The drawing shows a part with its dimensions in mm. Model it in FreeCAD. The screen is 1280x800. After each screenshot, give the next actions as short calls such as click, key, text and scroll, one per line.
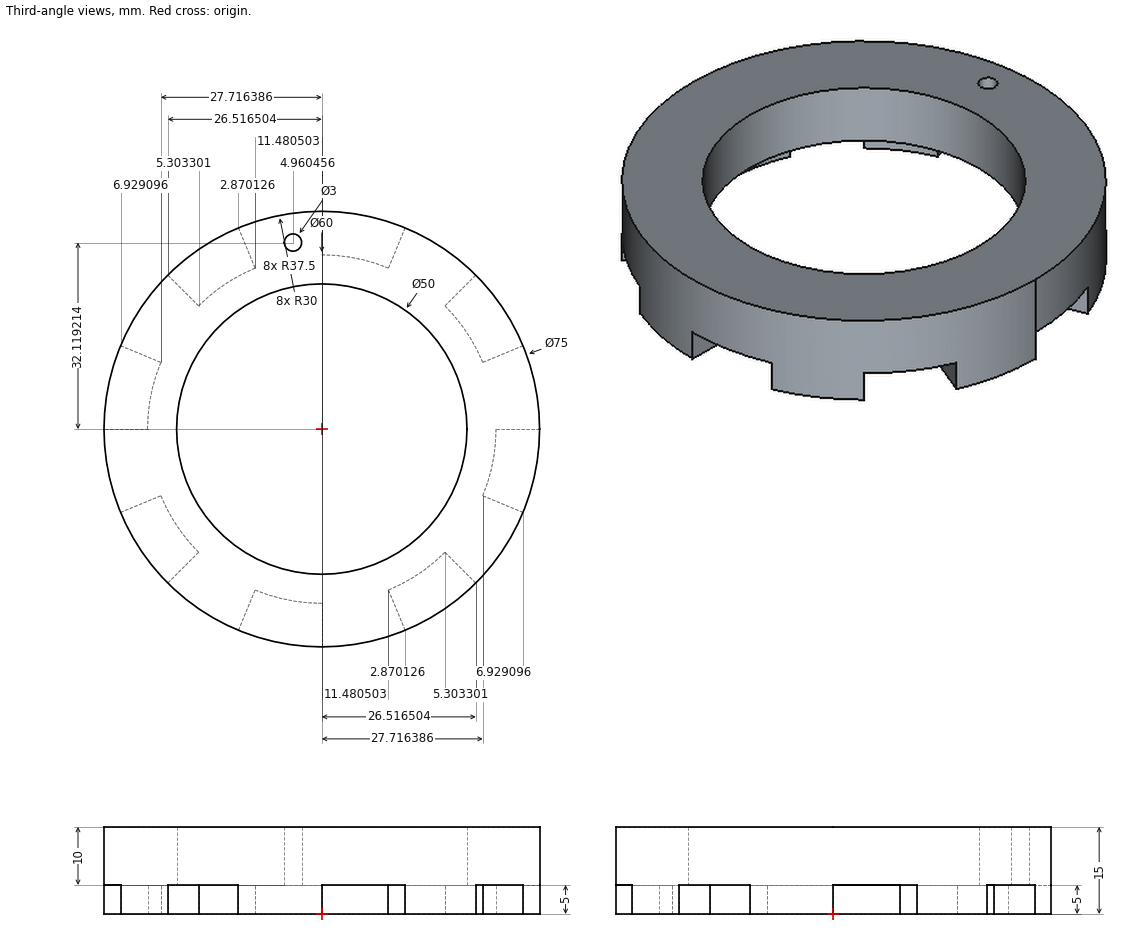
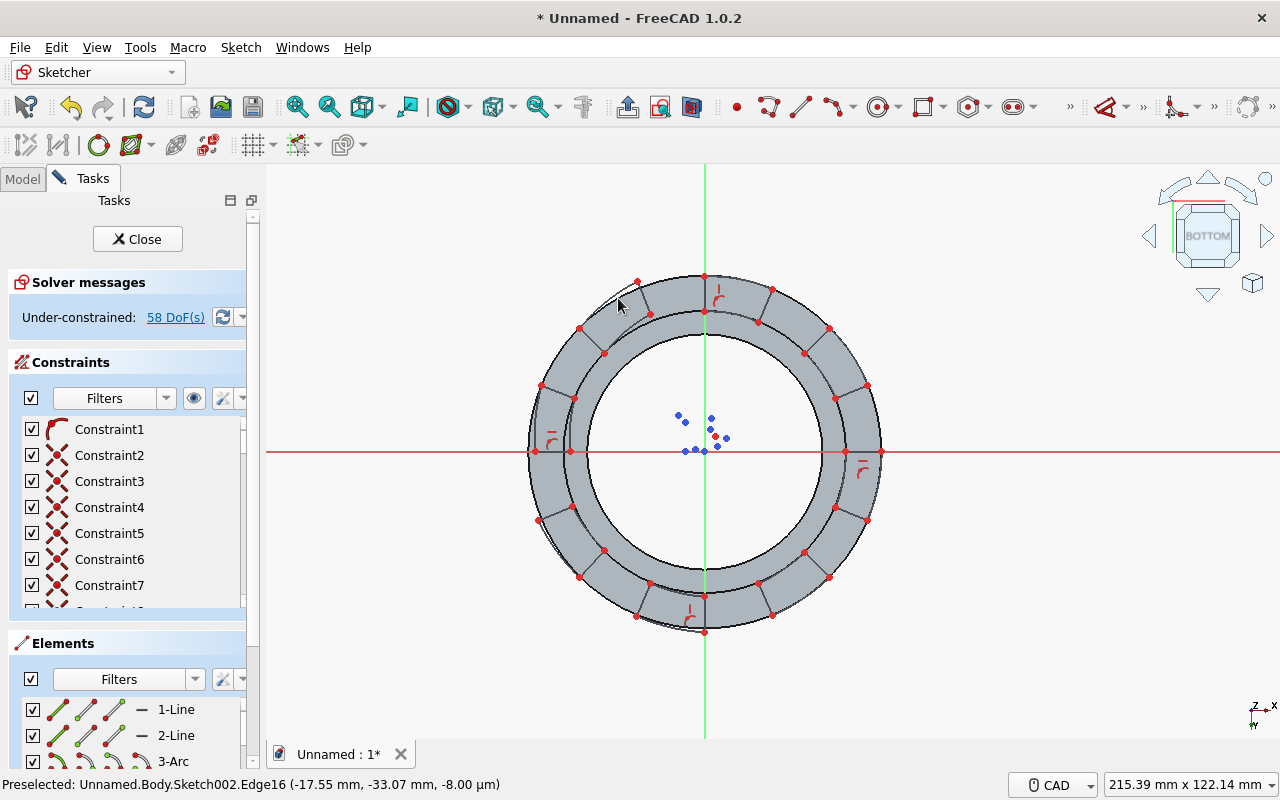
click(666, 589)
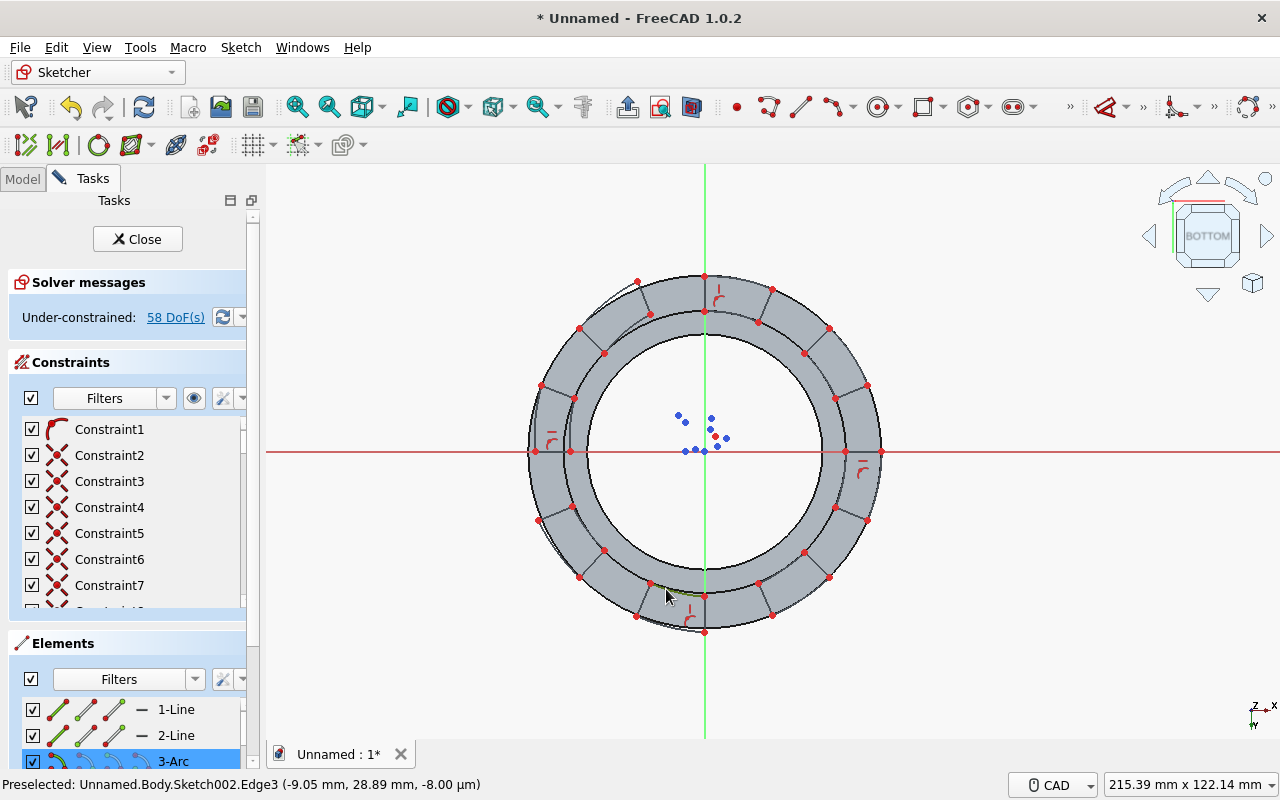
click(743, 316)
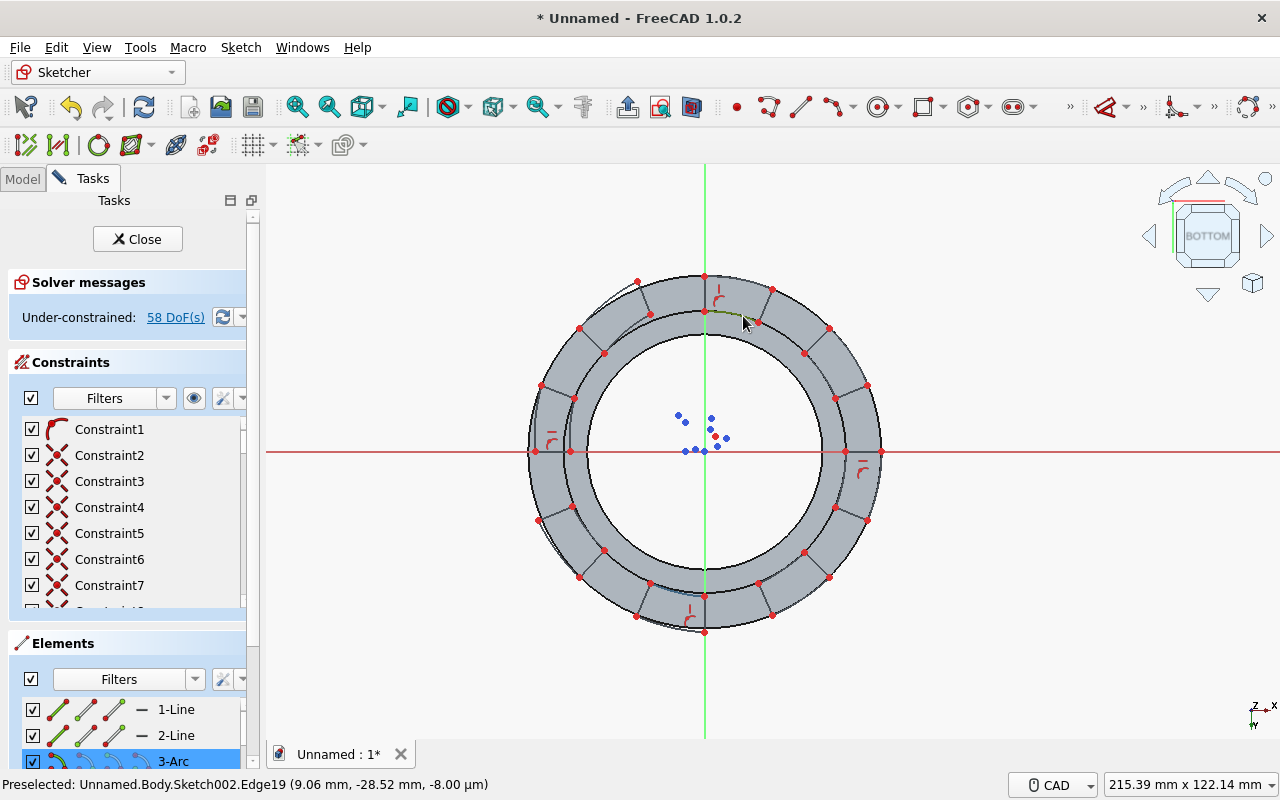
key(c)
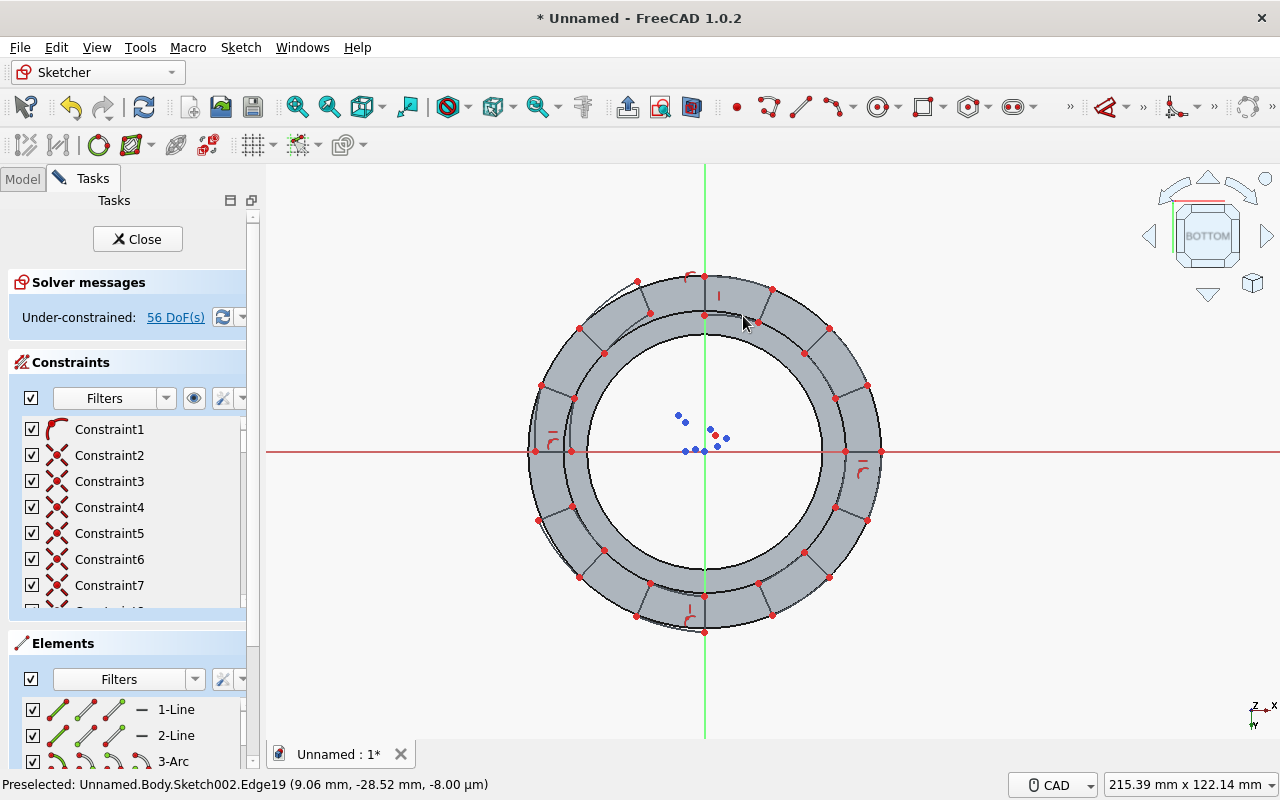
click(666, 589)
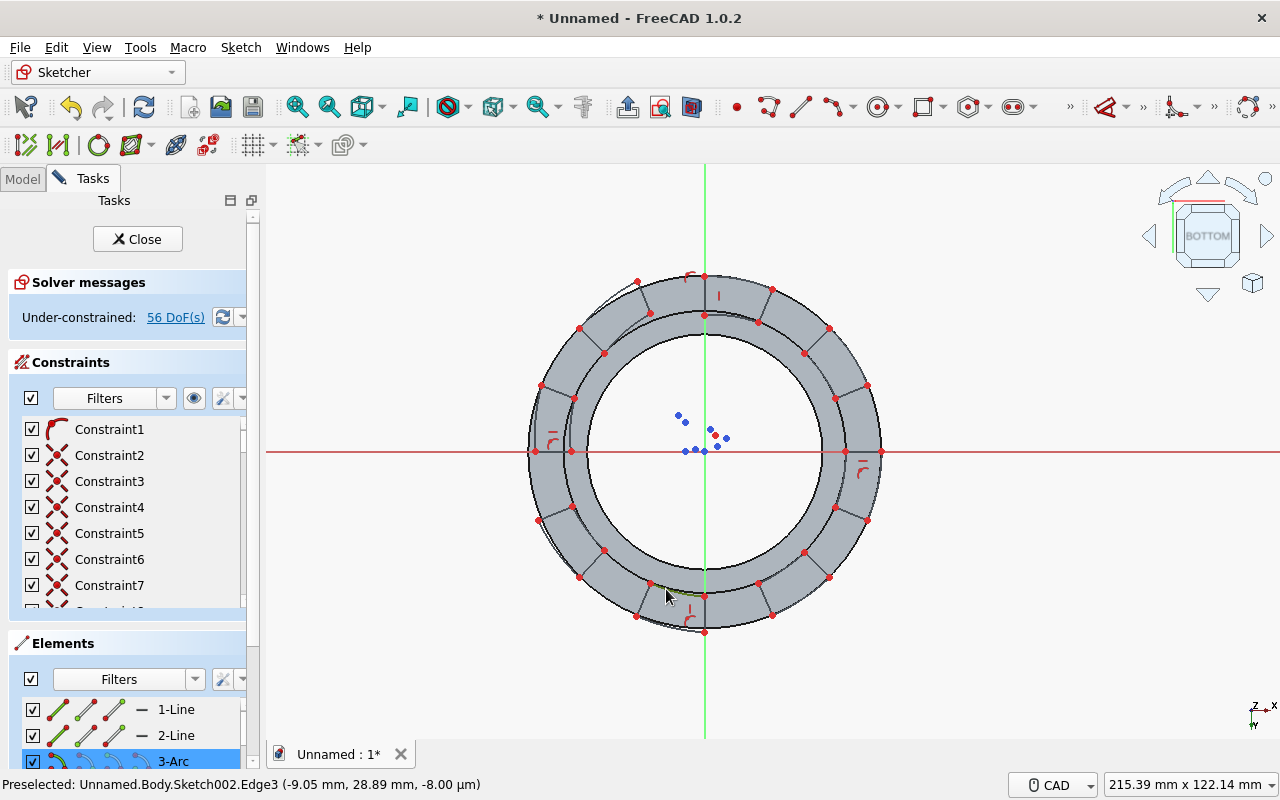
click(753, 282)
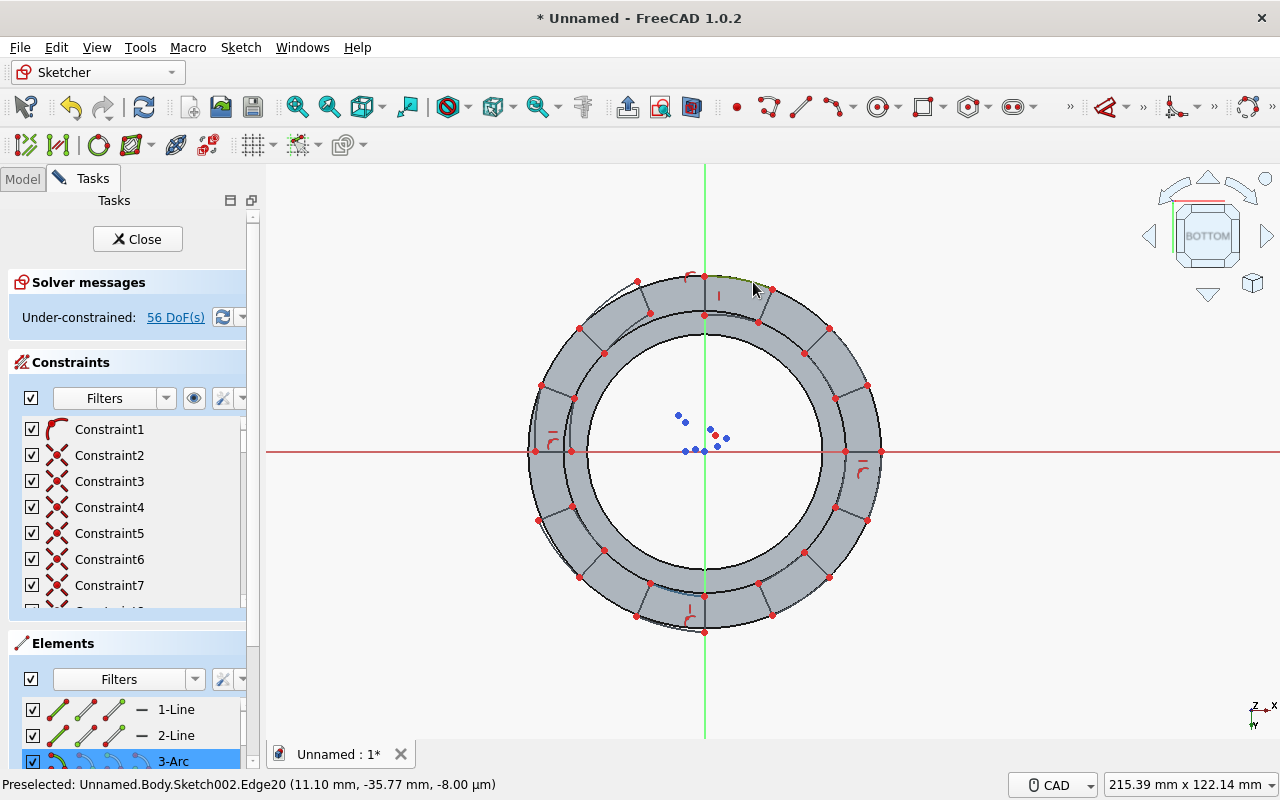
key(c)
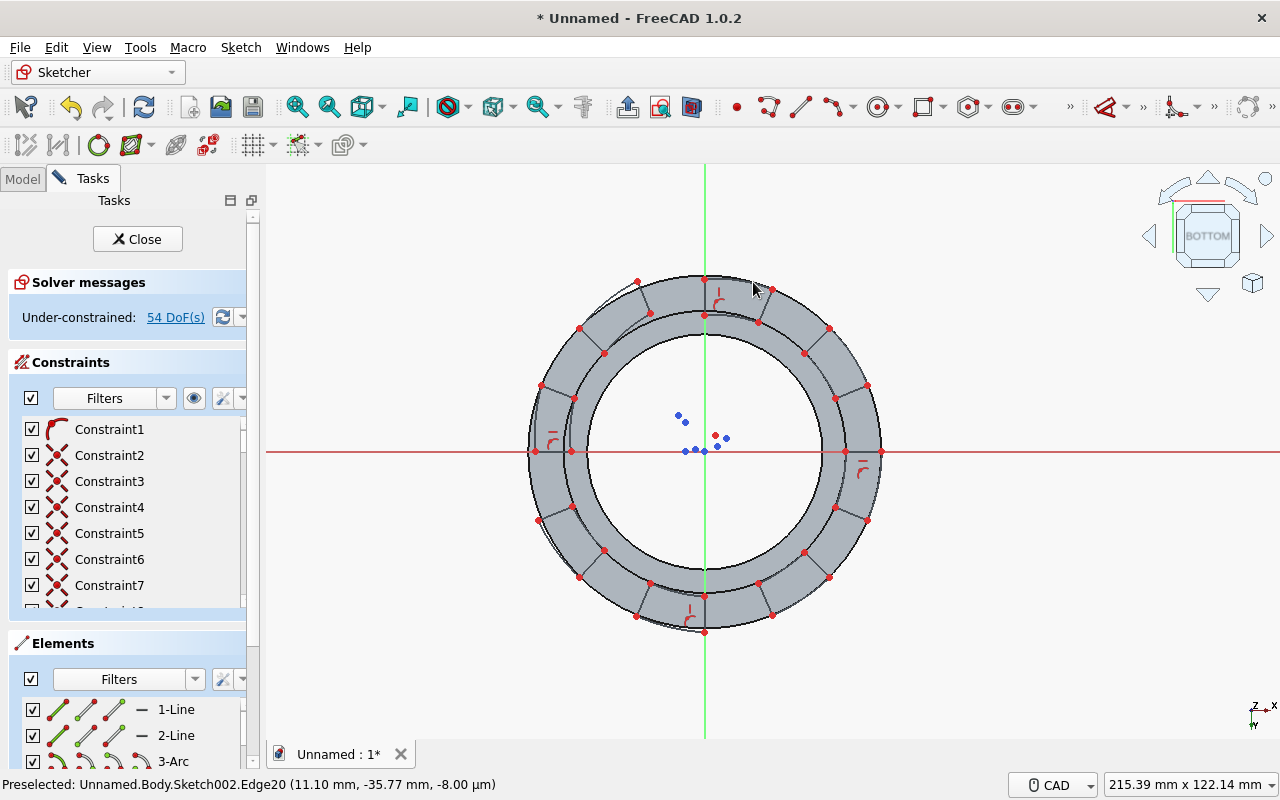
click(666, 589)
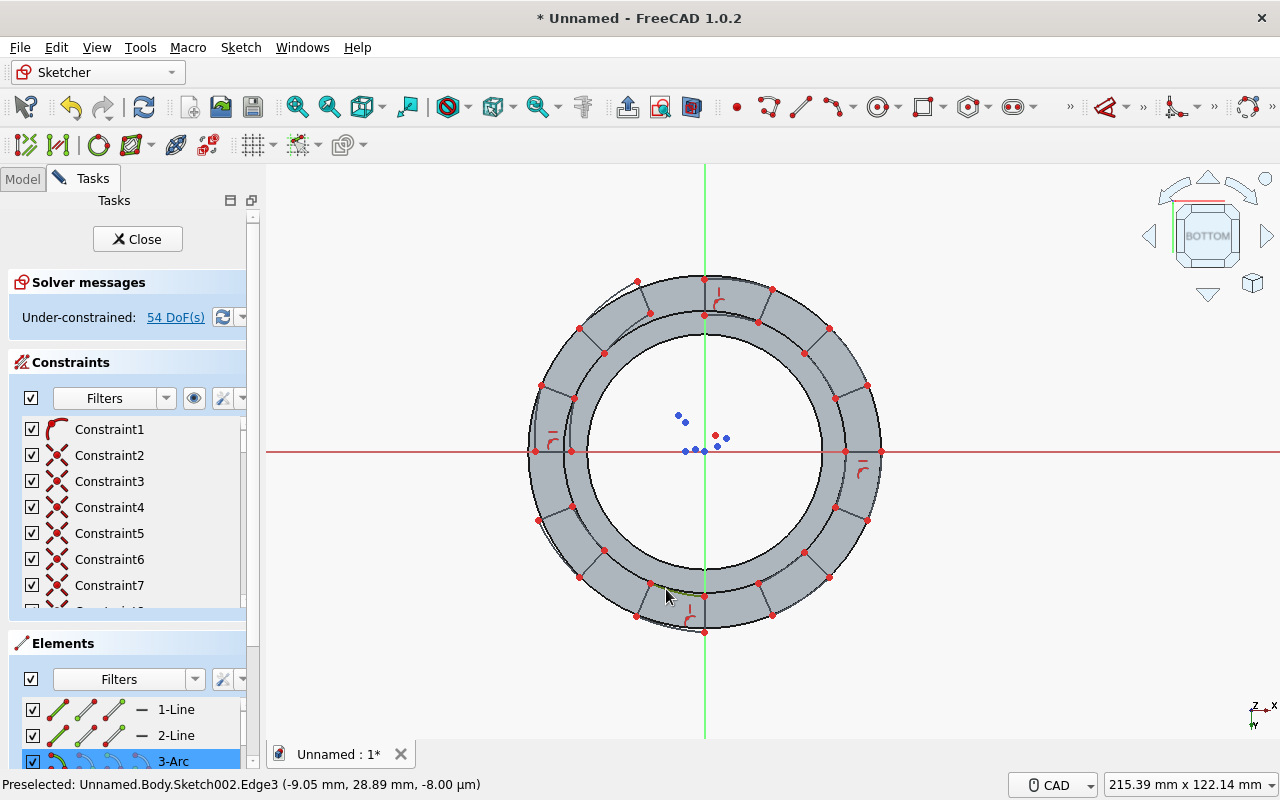
click(828, 384)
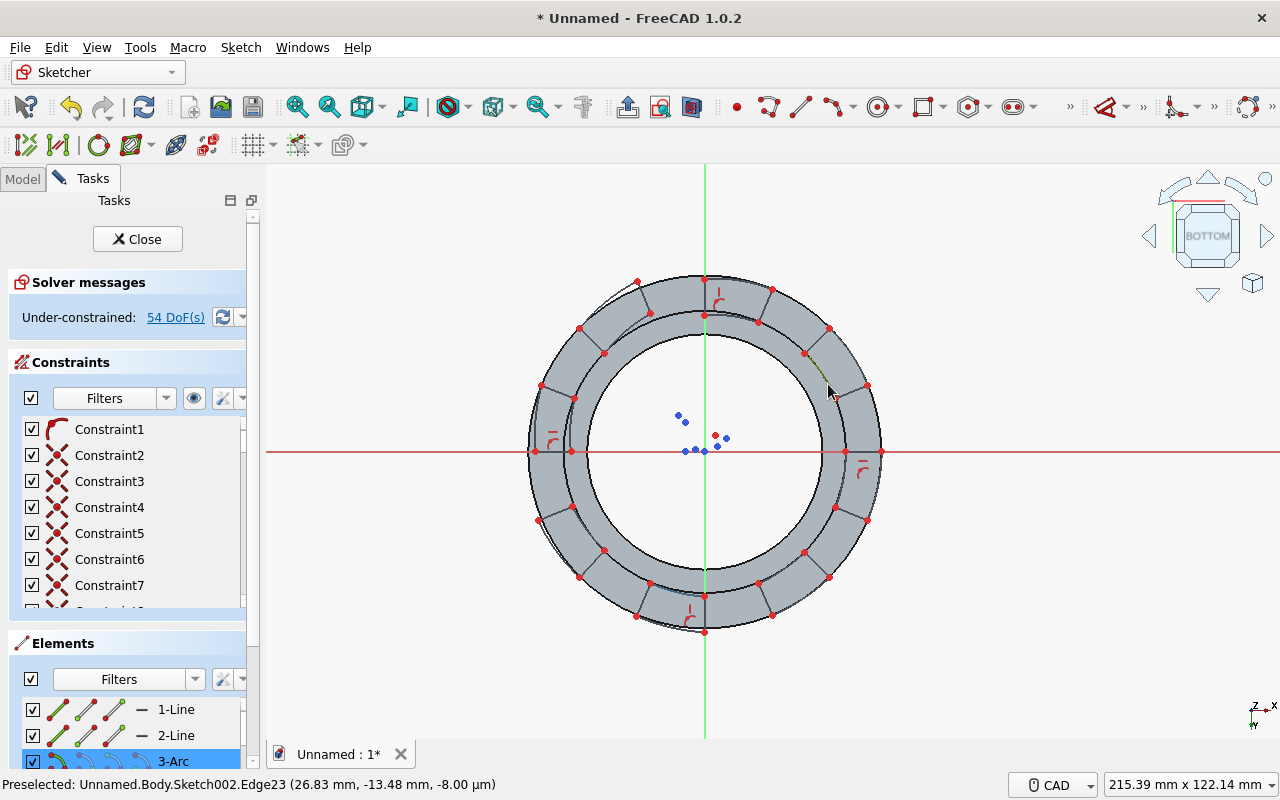
key(c)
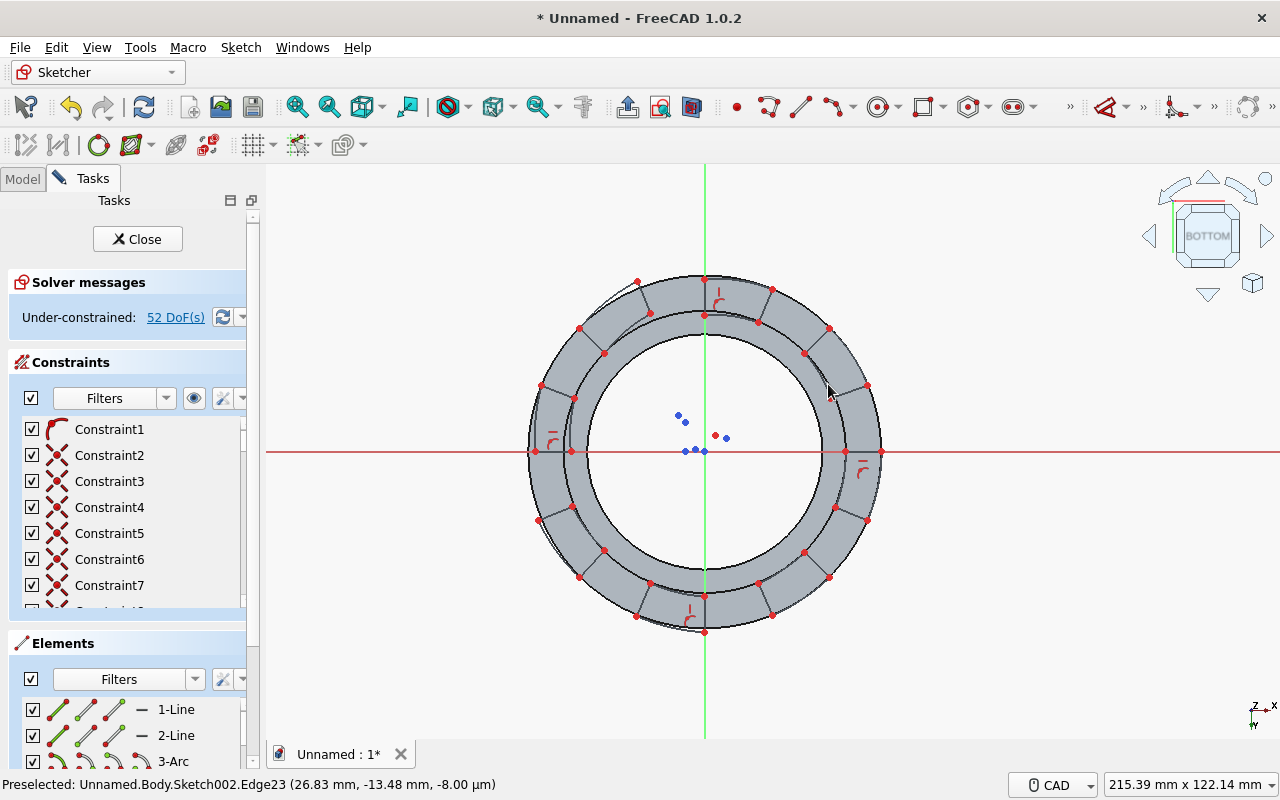
click(666, 589)